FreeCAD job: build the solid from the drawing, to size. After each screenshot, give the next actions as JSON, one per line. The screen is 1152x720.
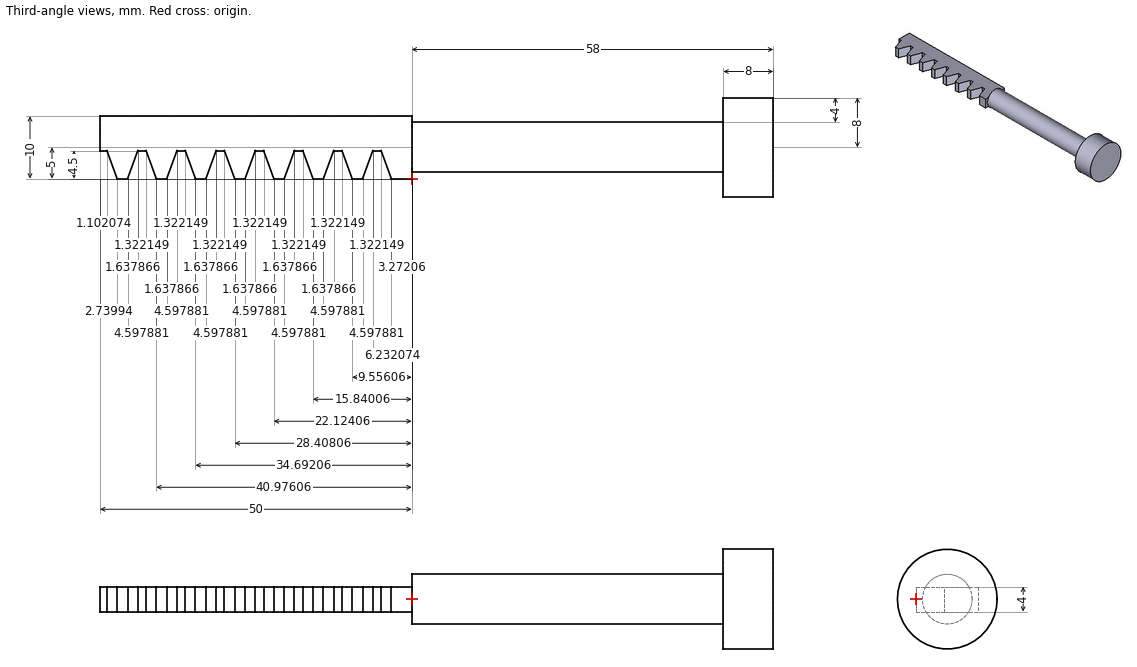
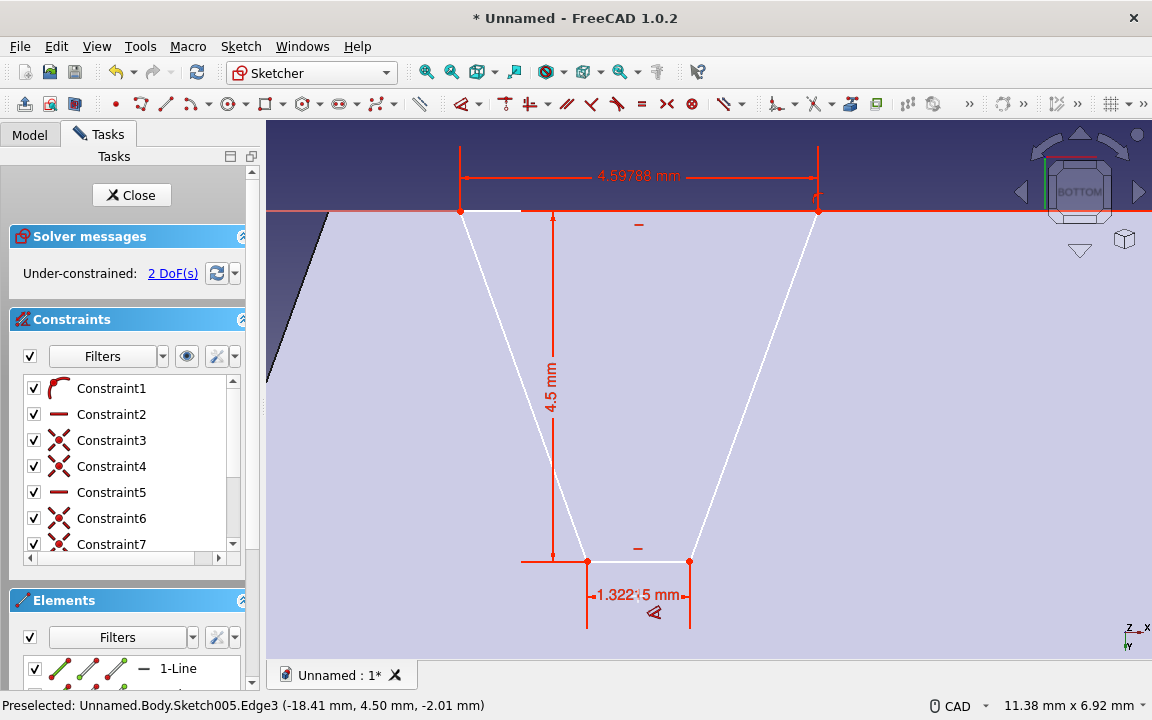
{"action": "left_click", "coordinate": [818, 211]}
{"action": "left_click", "coordinate": [903, 177]}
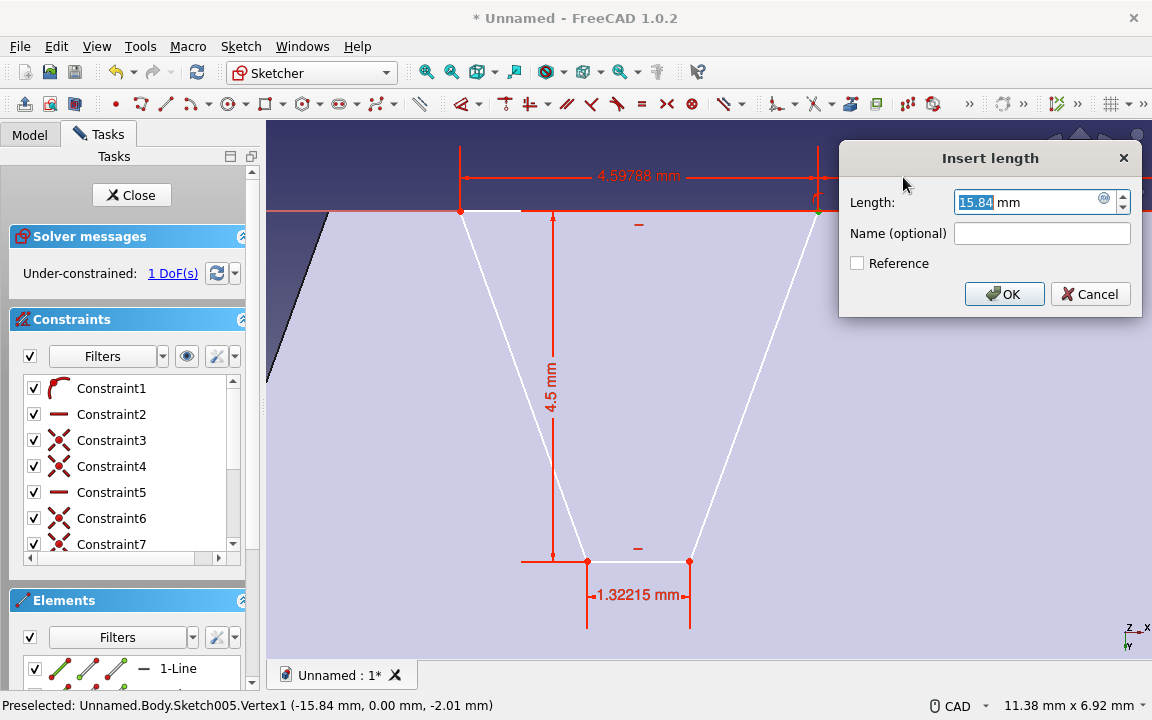
{"action": "type", "text": "15.84006"}
{"action": "key", "text": "Return"}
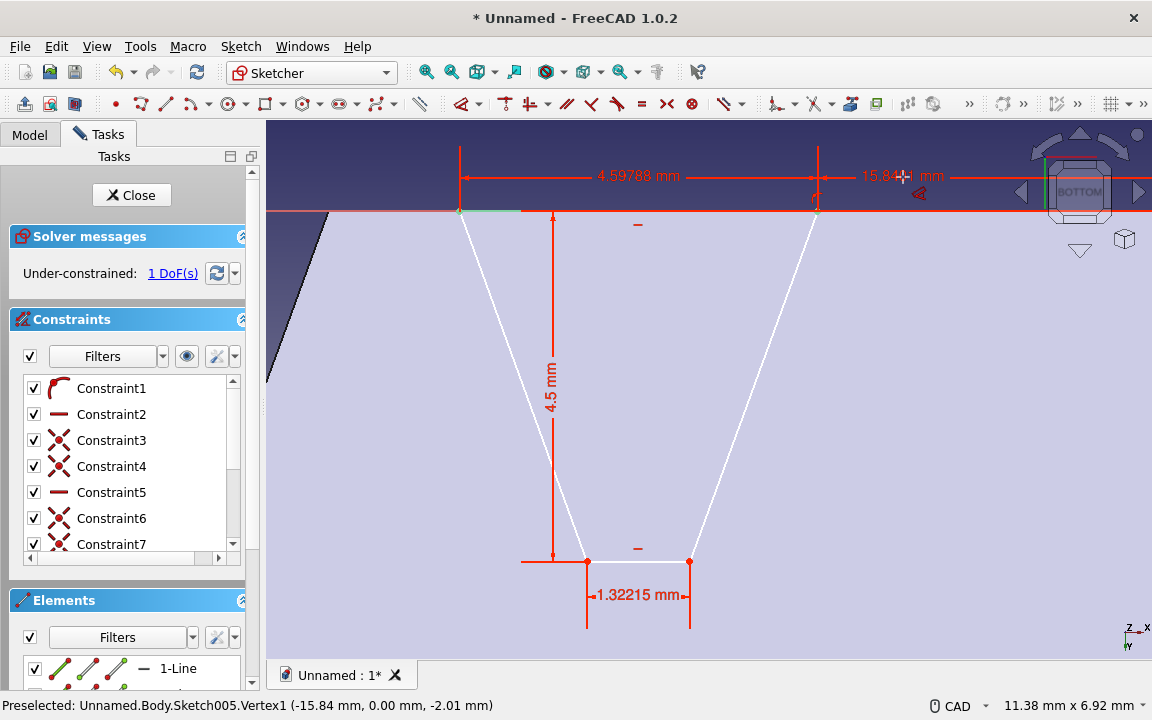
{"action": "left_click", "coordinate": [498, 317]}
{"action": "left_click", "coordinate": [523, 596]}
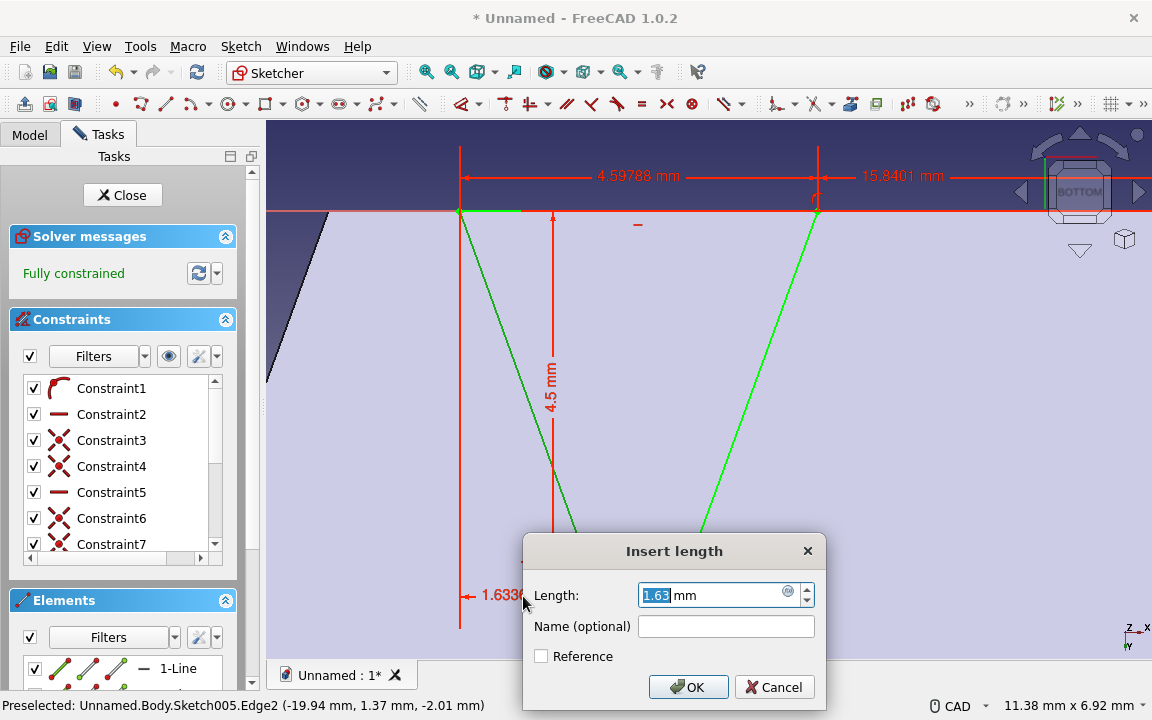
{"action": "type", "text": "1.637866"}
{"action": "key", "text": "Return"}
{"action": "key", "text": "Escape"}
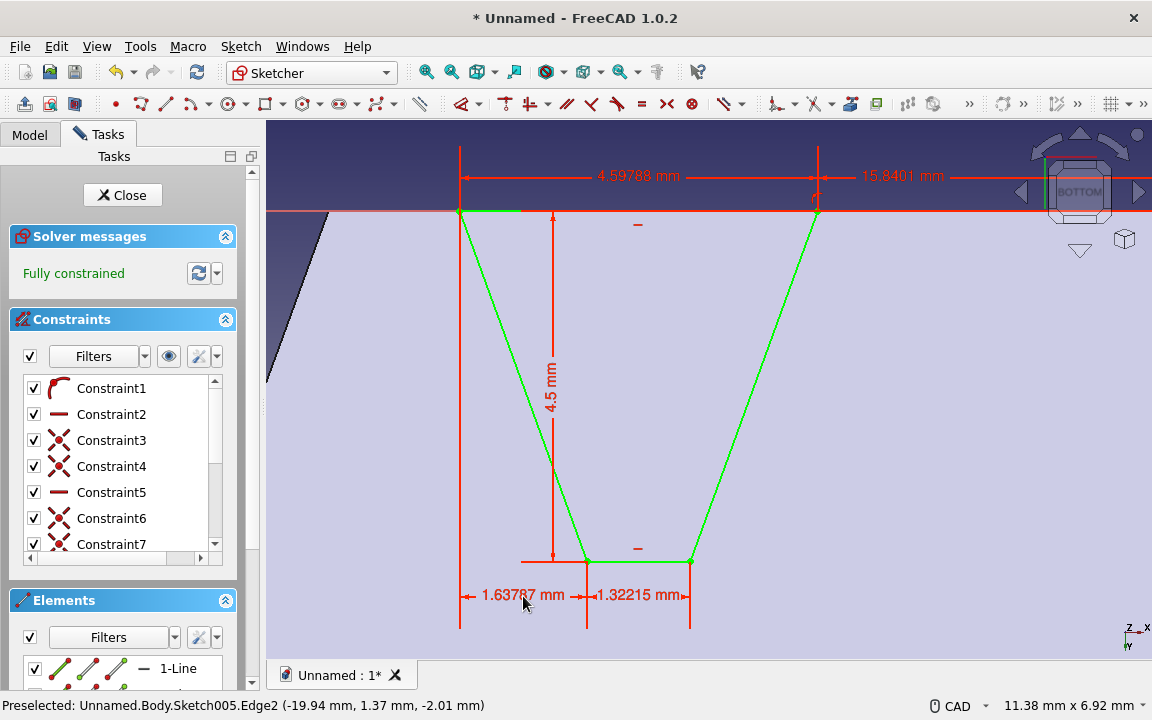
{"action": "left_click", "coordinate": [123, 195]}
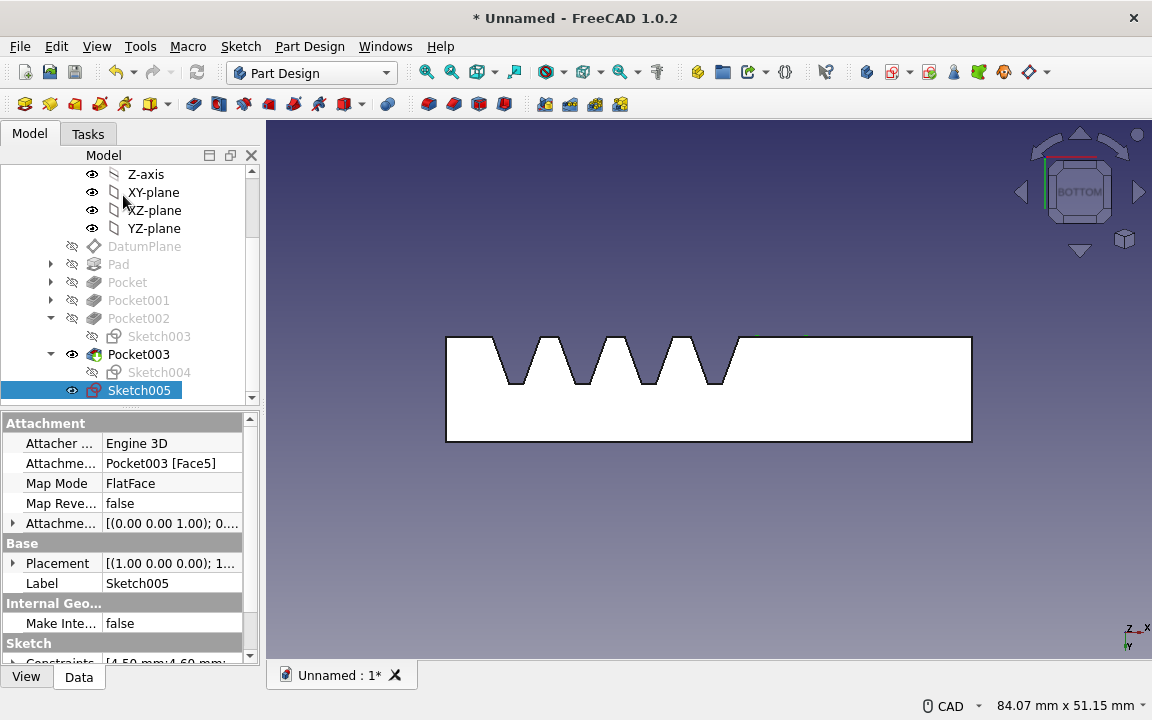
{"action": "left_click", "coordinate": [194, 104]}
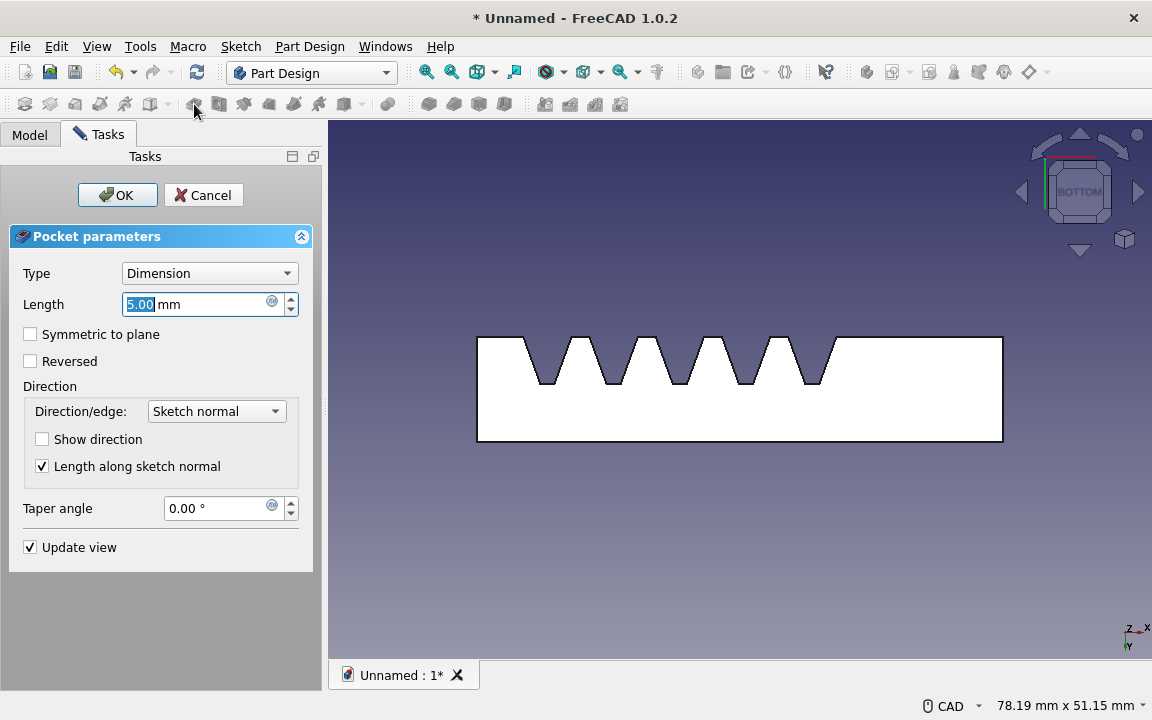
{"action": "left_click", "coordinate": [210, 274]}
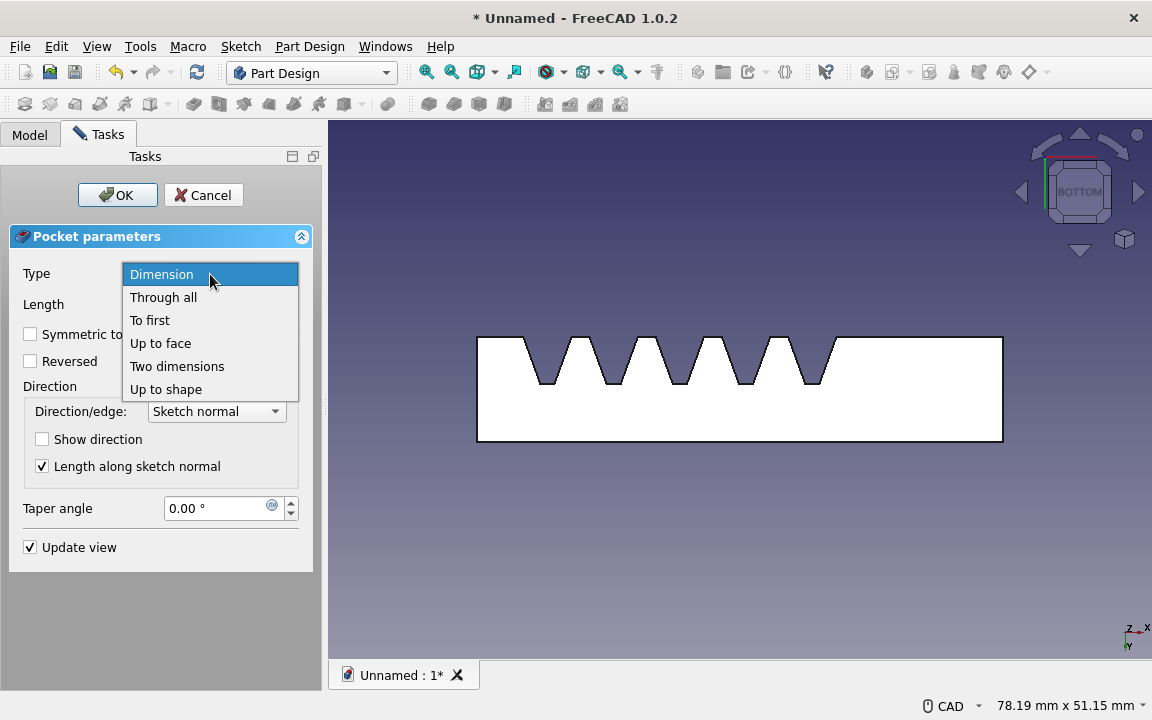
{"action": "left_click", "coordinate": [208, 298]}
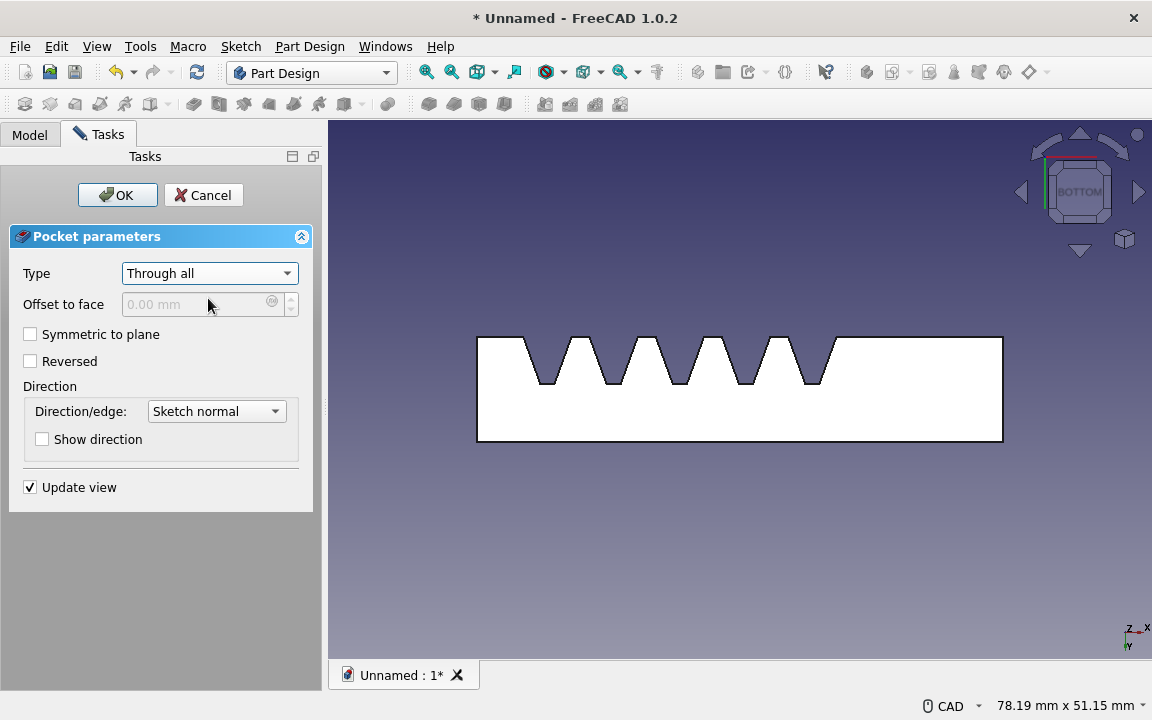
{"action": "left_click", "coordinate": [118, 195]}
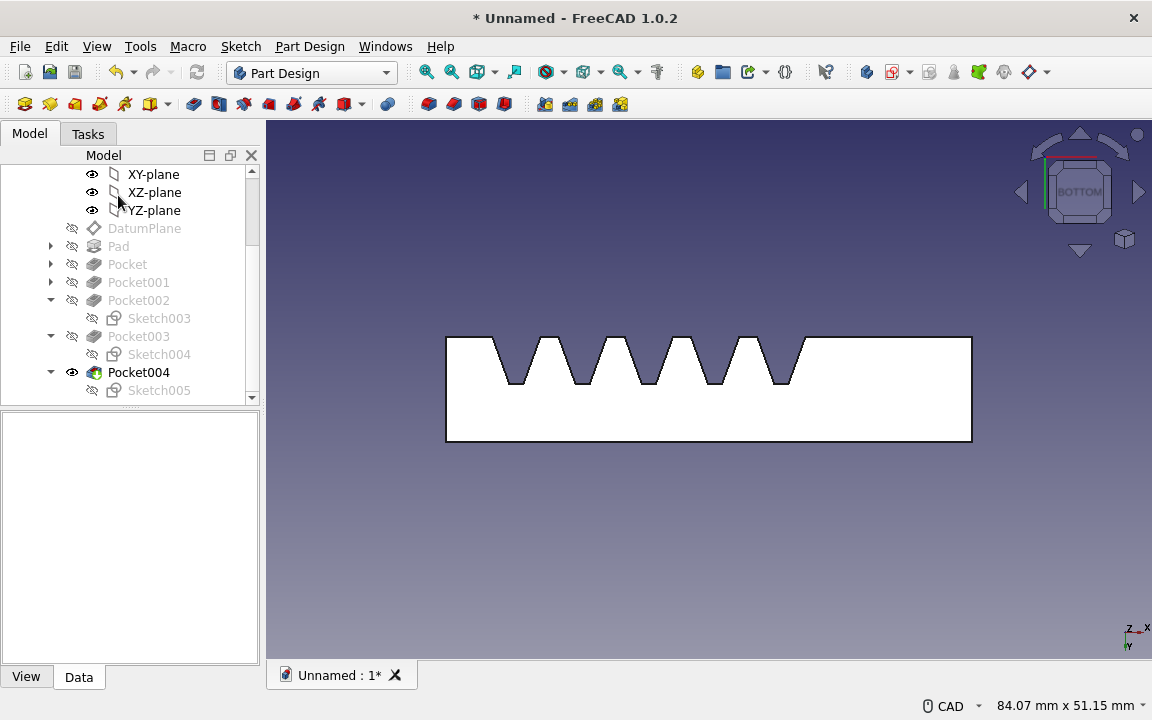
{"action": "left_click", "coordinate": [860, 389]}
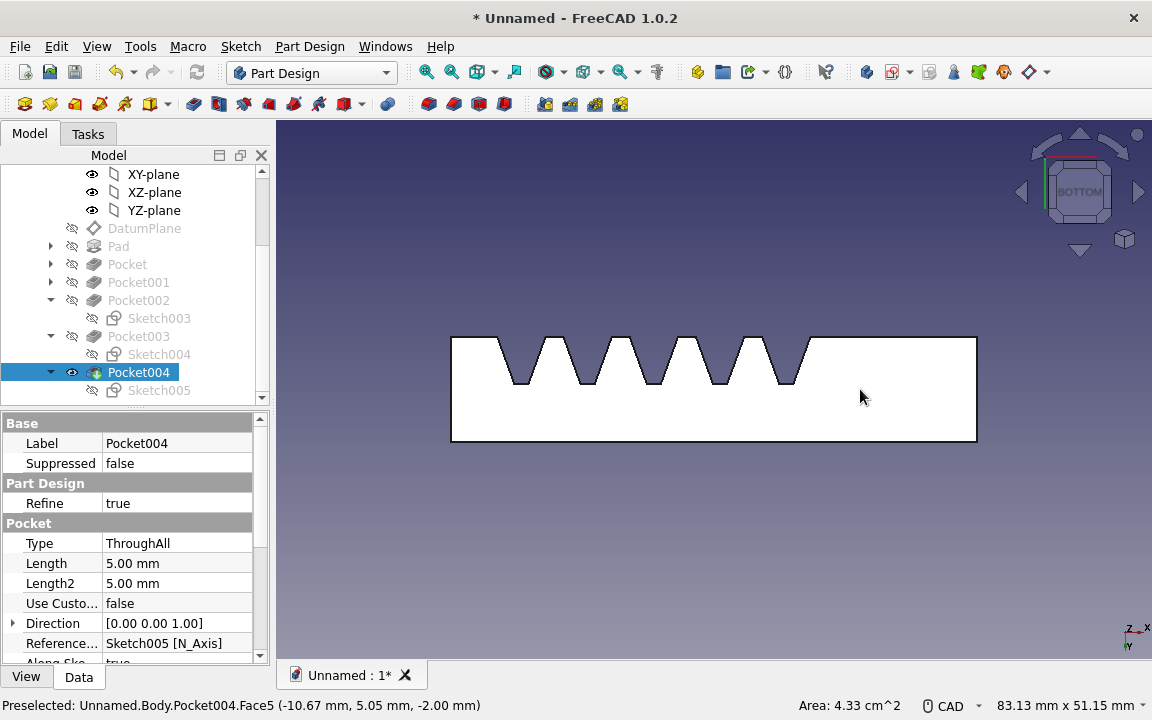
{"action": "left_click", "coordinate": [892, 72]}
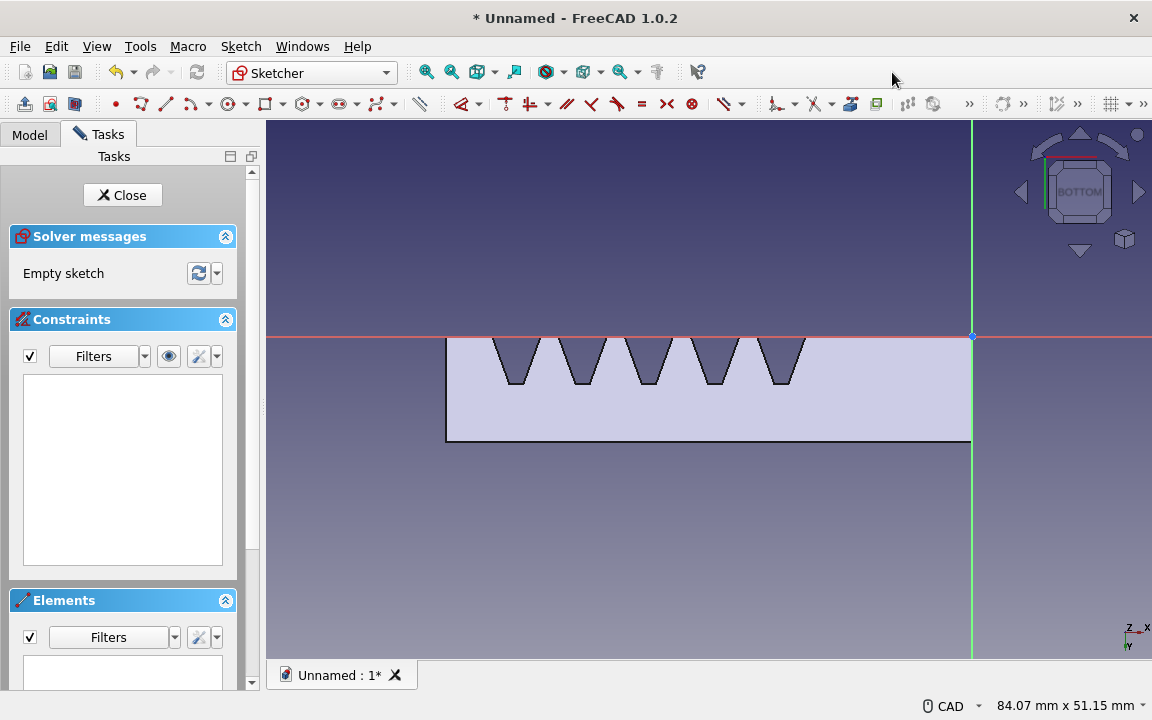
{"action": "scroll", "coordinate": [880, 356], "scroll_direction": "up", "scroll_amount": 10}